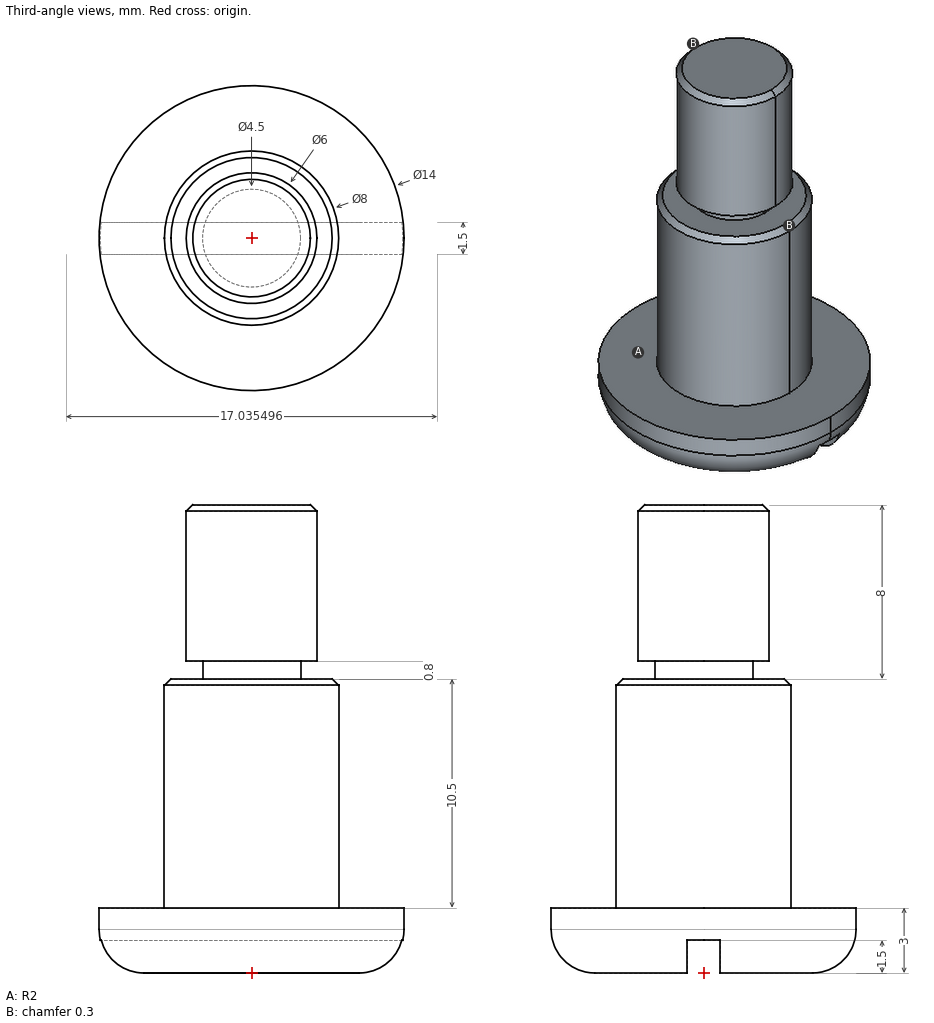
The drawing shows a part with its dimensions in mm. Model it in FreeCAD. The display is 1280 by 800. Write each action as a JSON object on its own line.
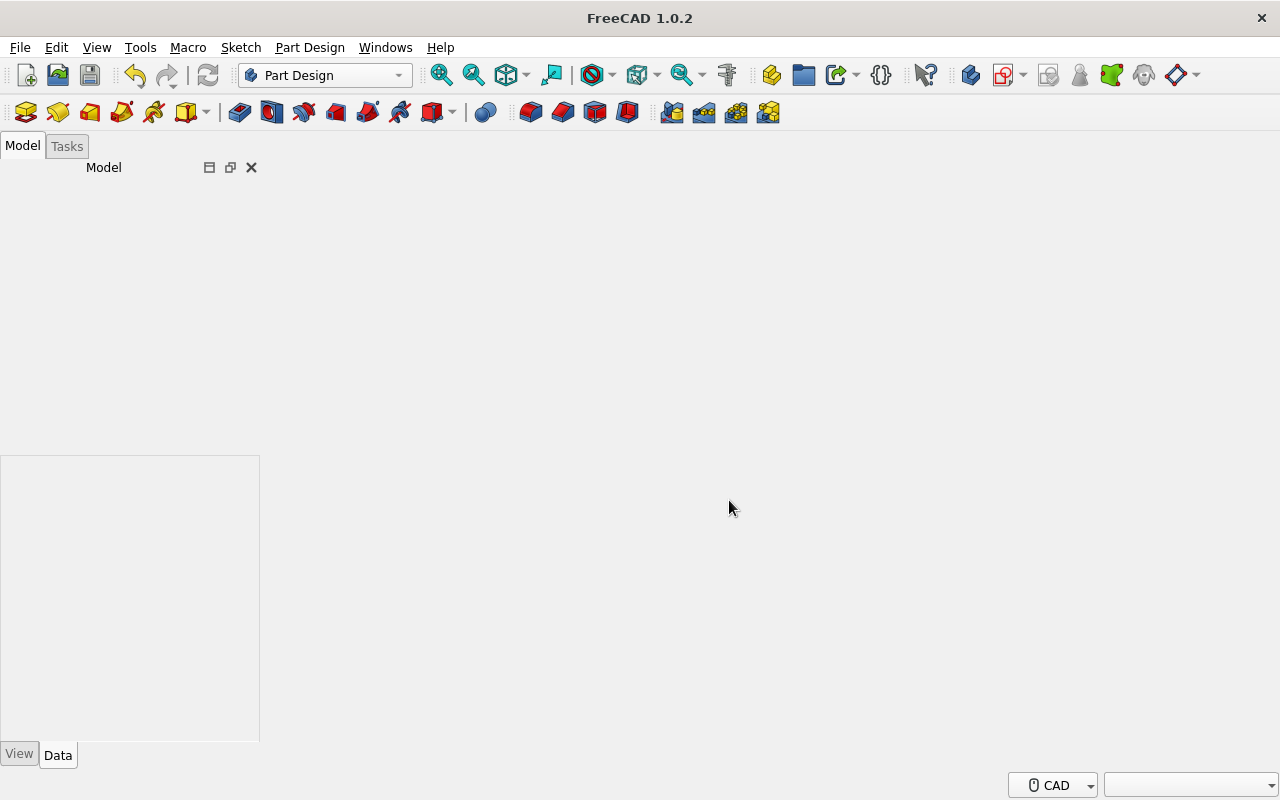
{"action": "left_click", "coordinate": [26, 76]}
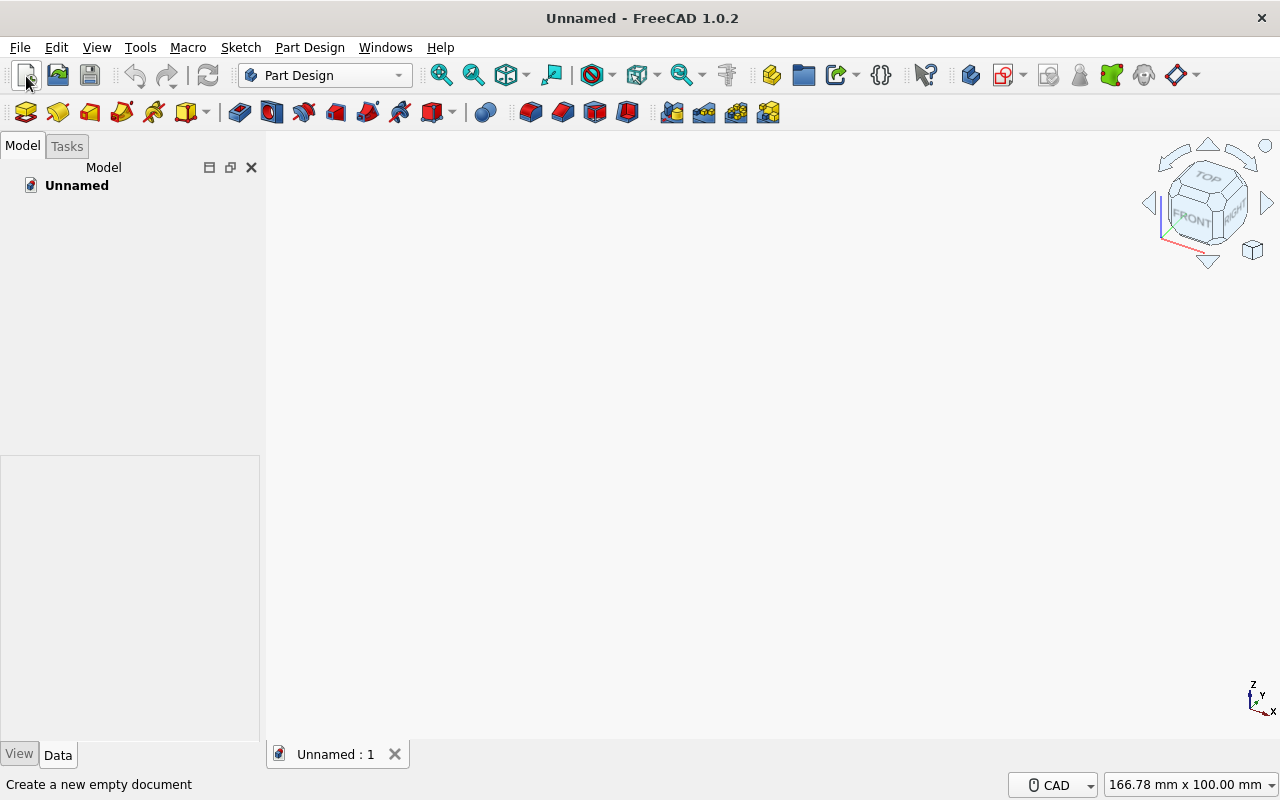
{"action": "left_click", "coordinate": [1004, 76]}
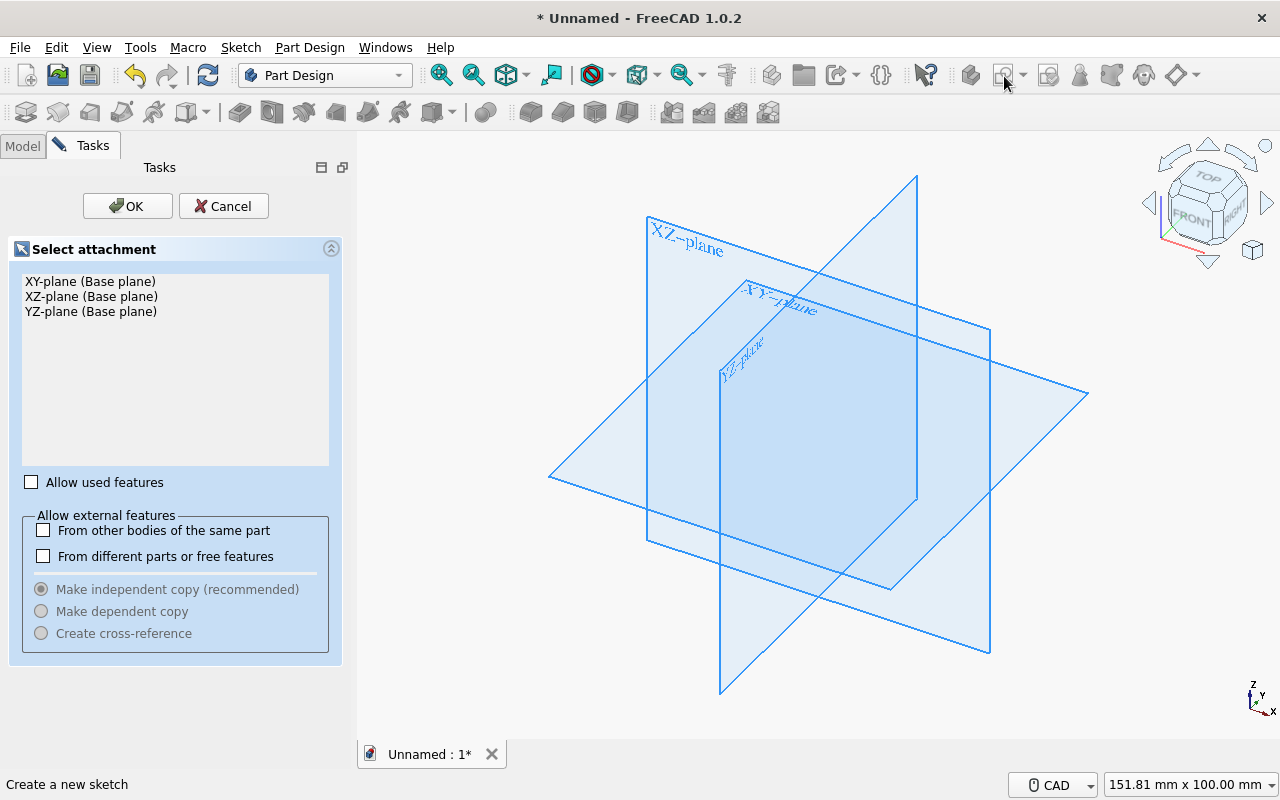
{"action": "left_click", "coordinate": [82, 282]}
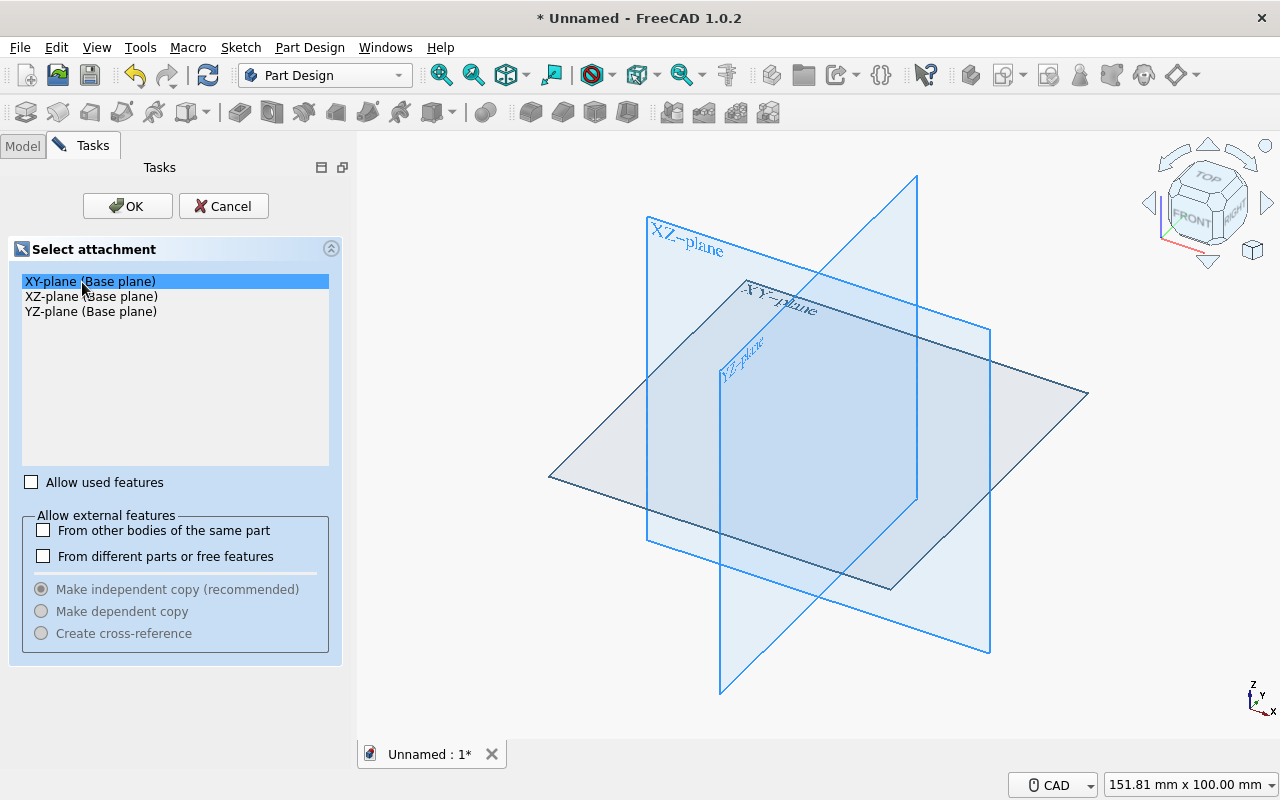
{"action": "left_click", "coordinate": [128, 206]}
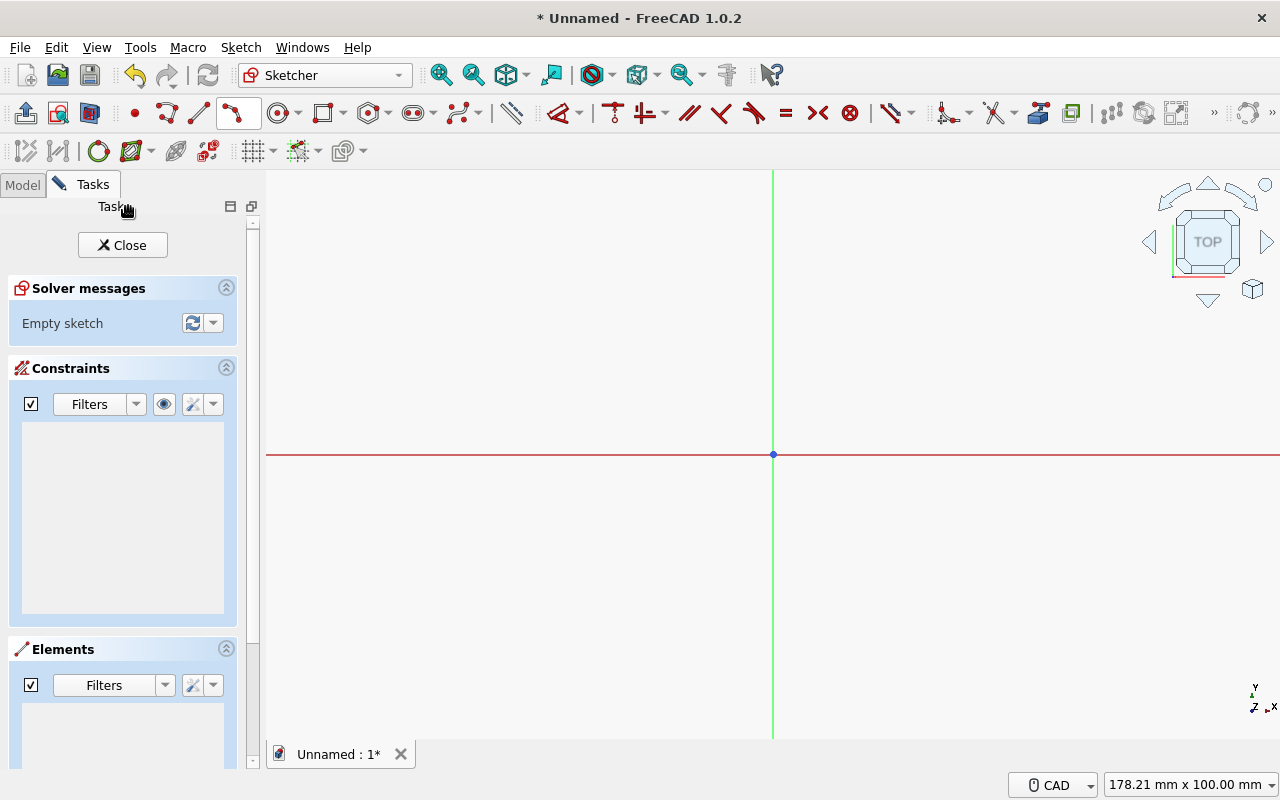
{"action": "scroll", "coordinate": [790, 454], "scroll_direction": "up", "scroll_amount": 8}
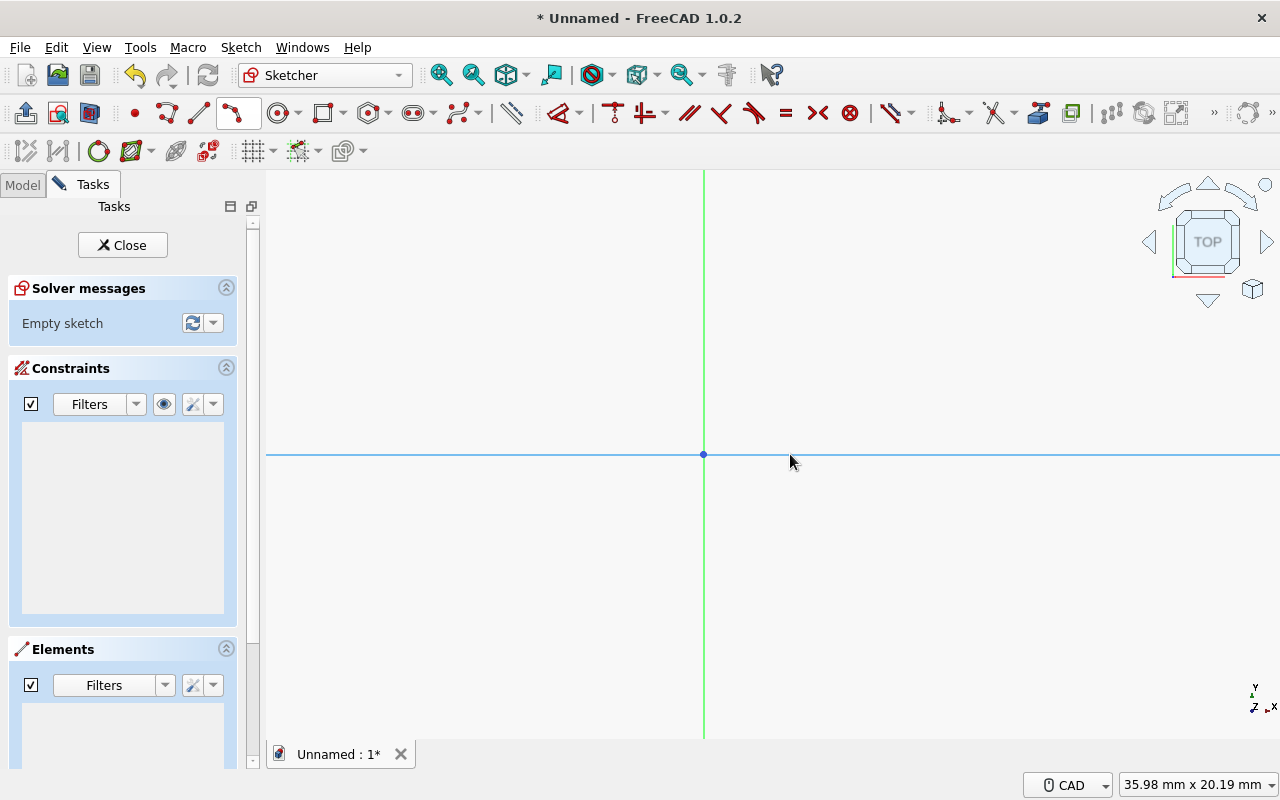
{"action": "left_click", "coordinate": [278, 114]}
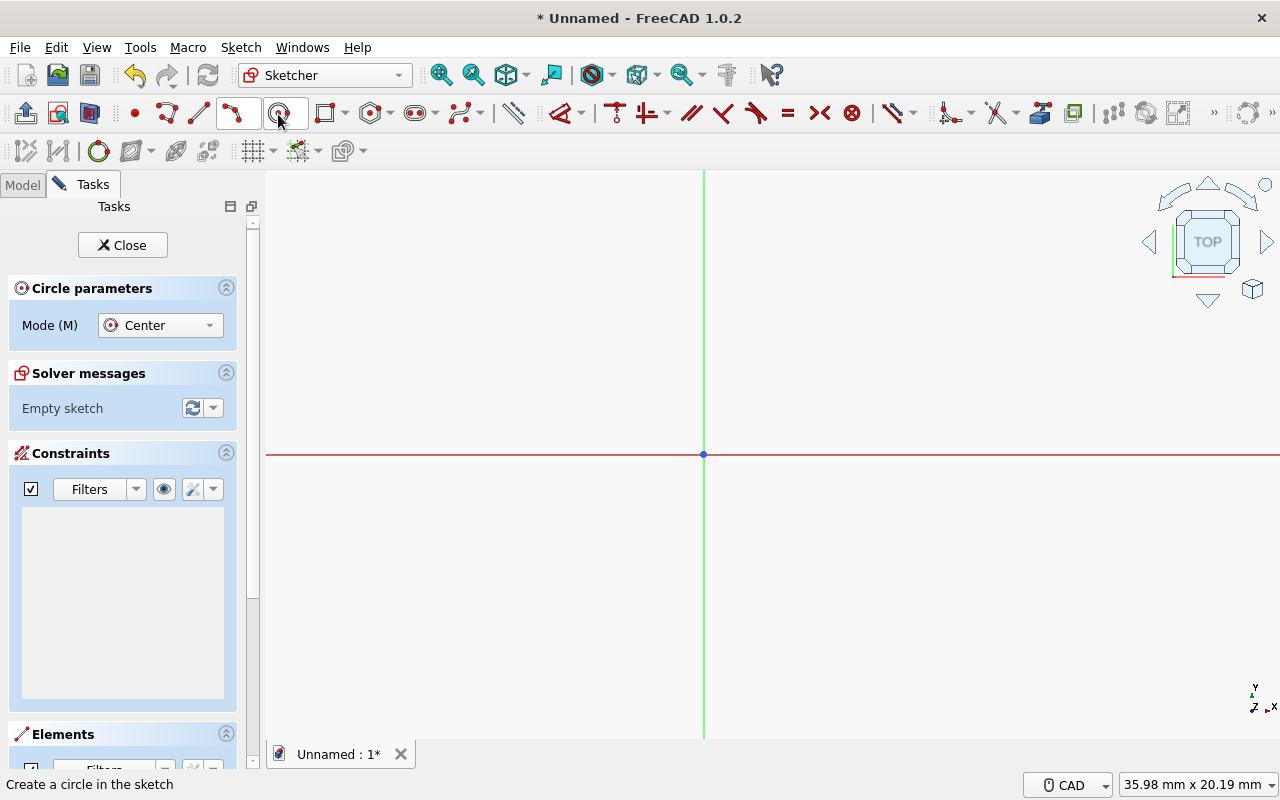
{"action": "left_click", "coordinate": [704, 454]}
{"action": "left_click", "coordinate": [843, 315]}
{"action": "key", "text": "Escape"}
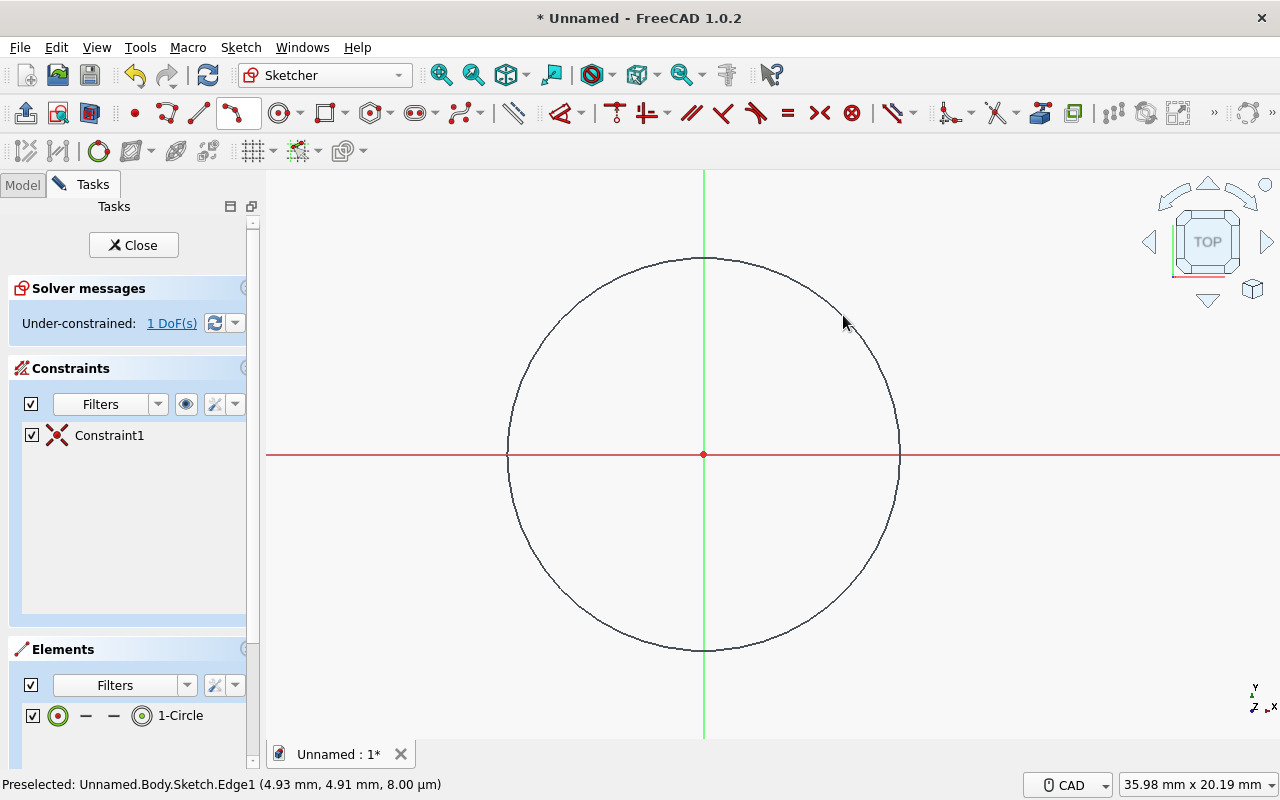
{"action": "left_click", "coordinate": [560, 114]}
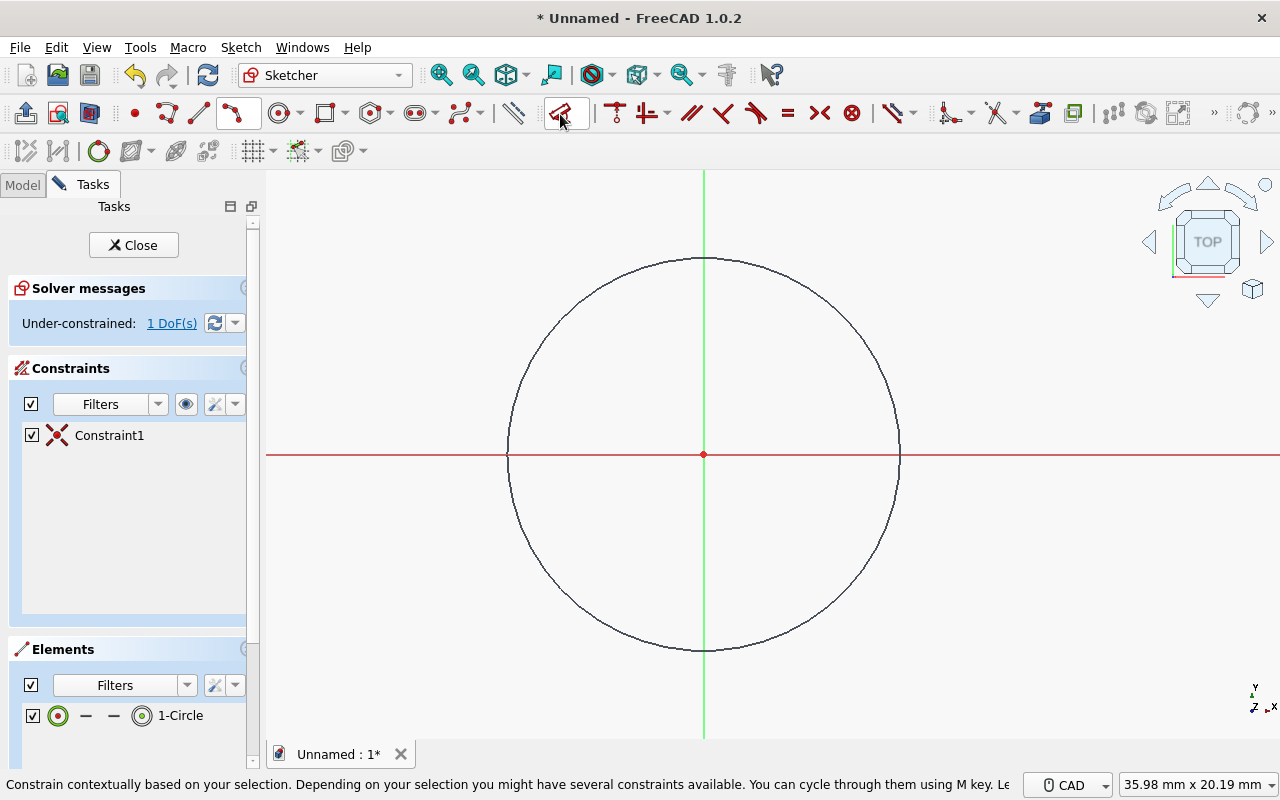
{"action": "left_click", "coordinate": [842, 315]}
{"action": "left_click", "coordinate": [865, 292]}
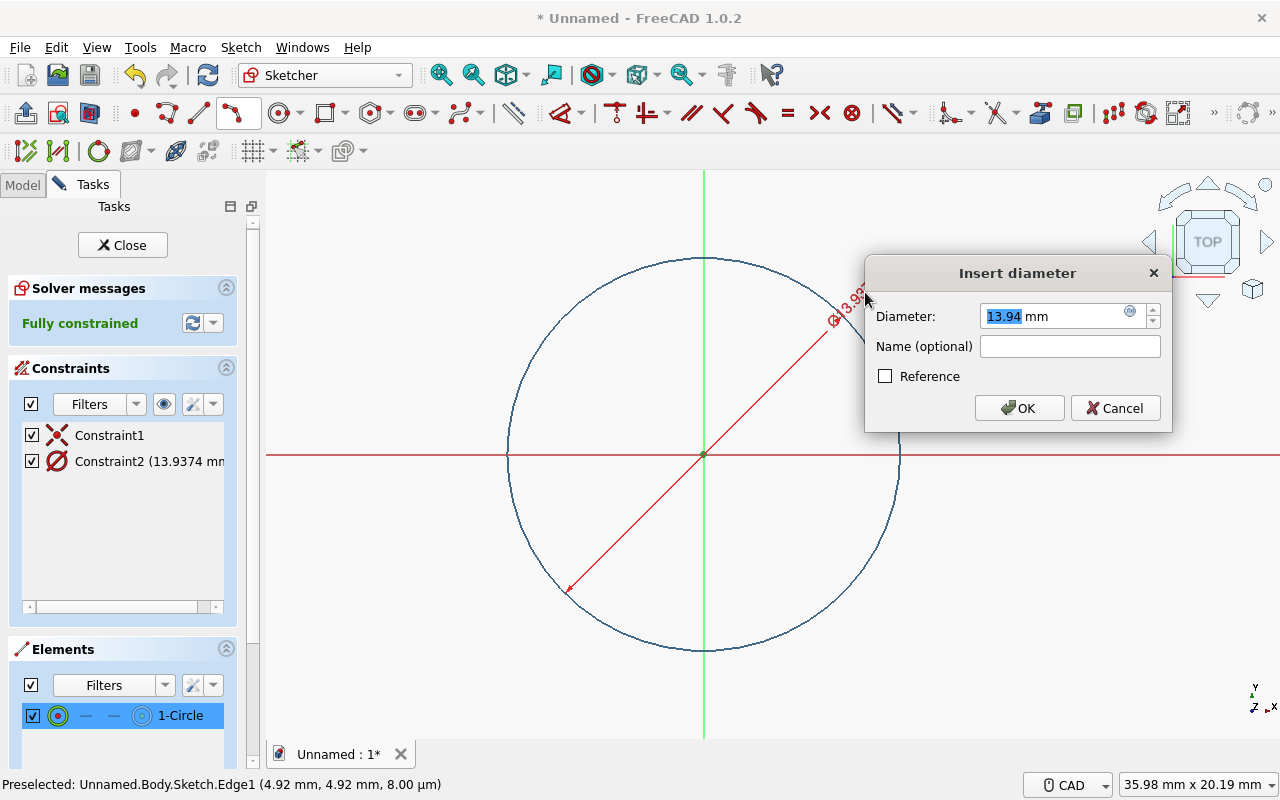
{"action": "type", "text": "14"}
{"action": "key", "text": "Return"}
{"action": "key", "text": "Escape"}